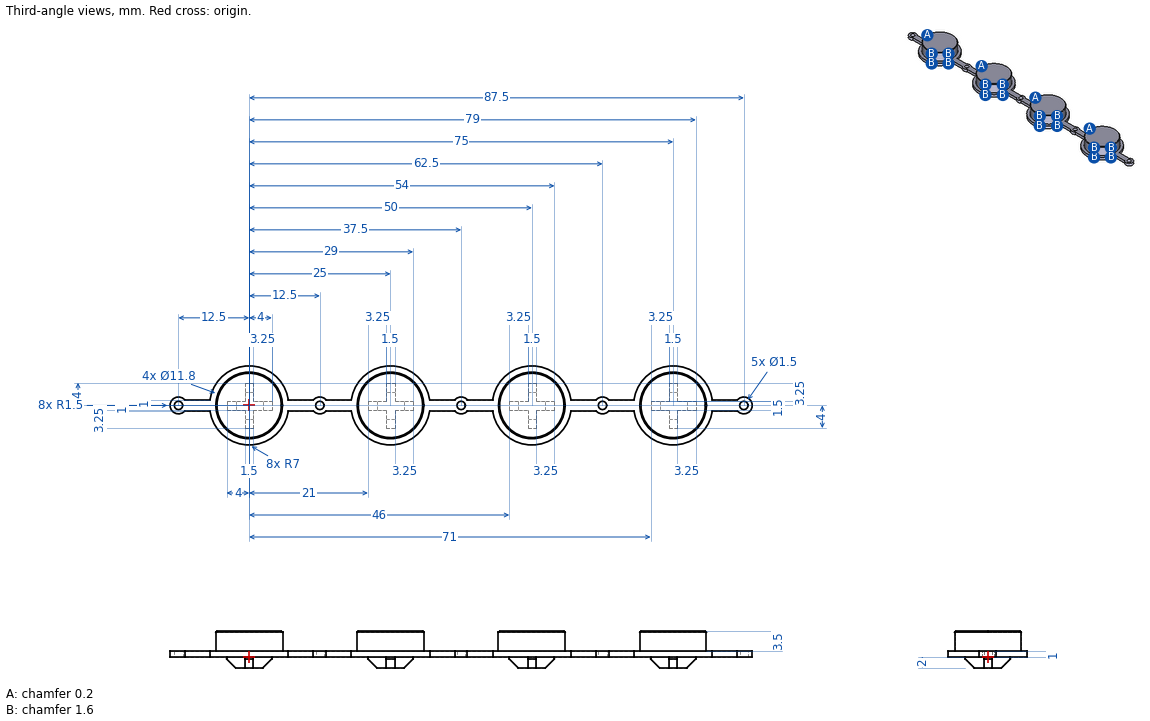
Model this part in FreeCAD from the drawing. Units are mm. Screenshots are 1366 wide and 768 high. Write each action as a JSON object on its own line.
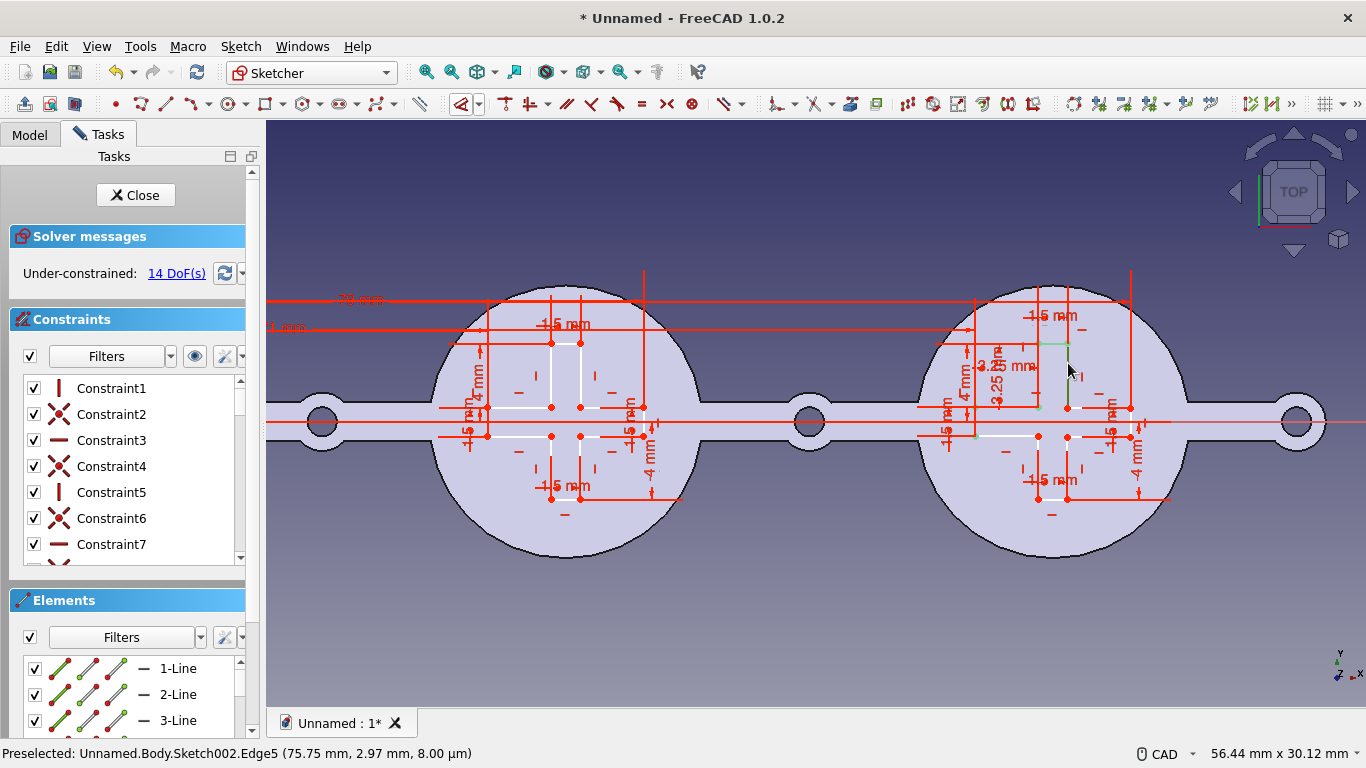
{"action": "key", "text": "i"}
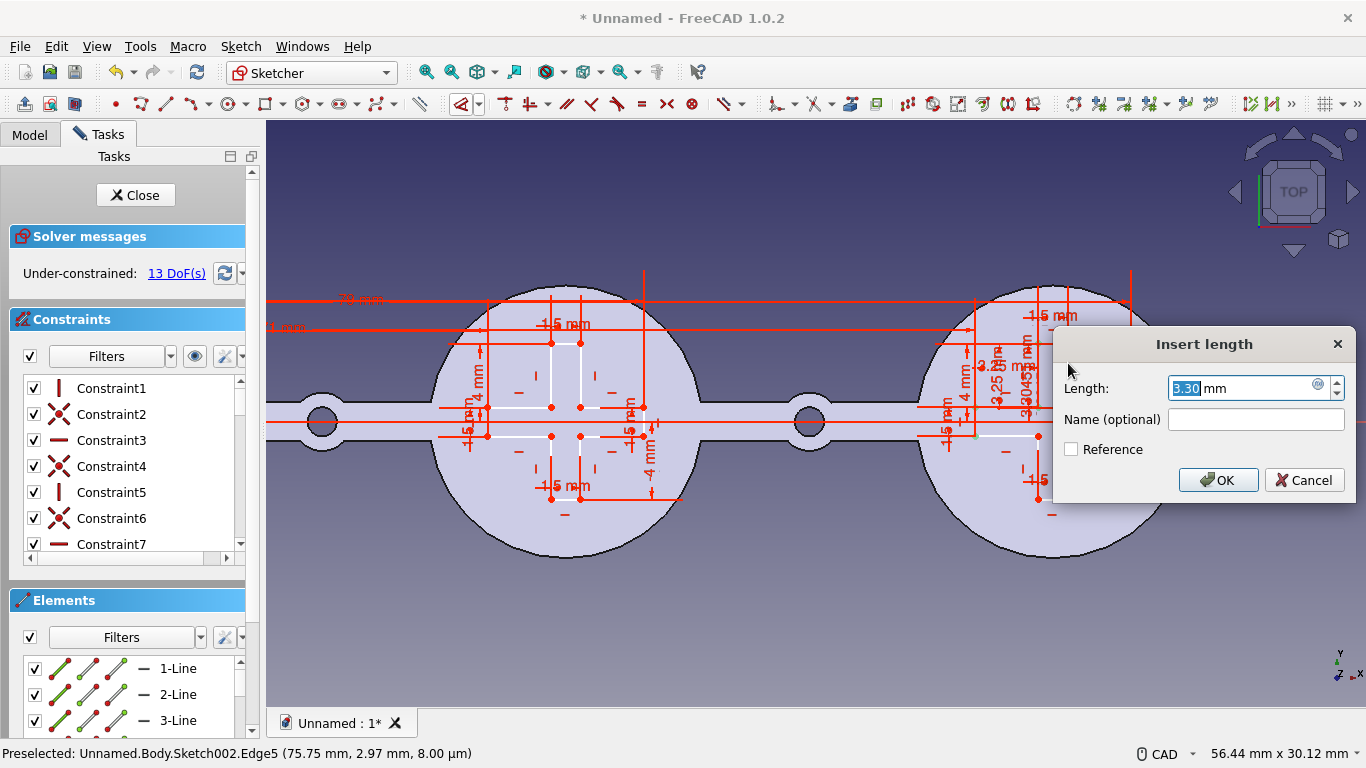
{"action": "type", "text": "3.25"}
{"action": "key", "text": "Return"}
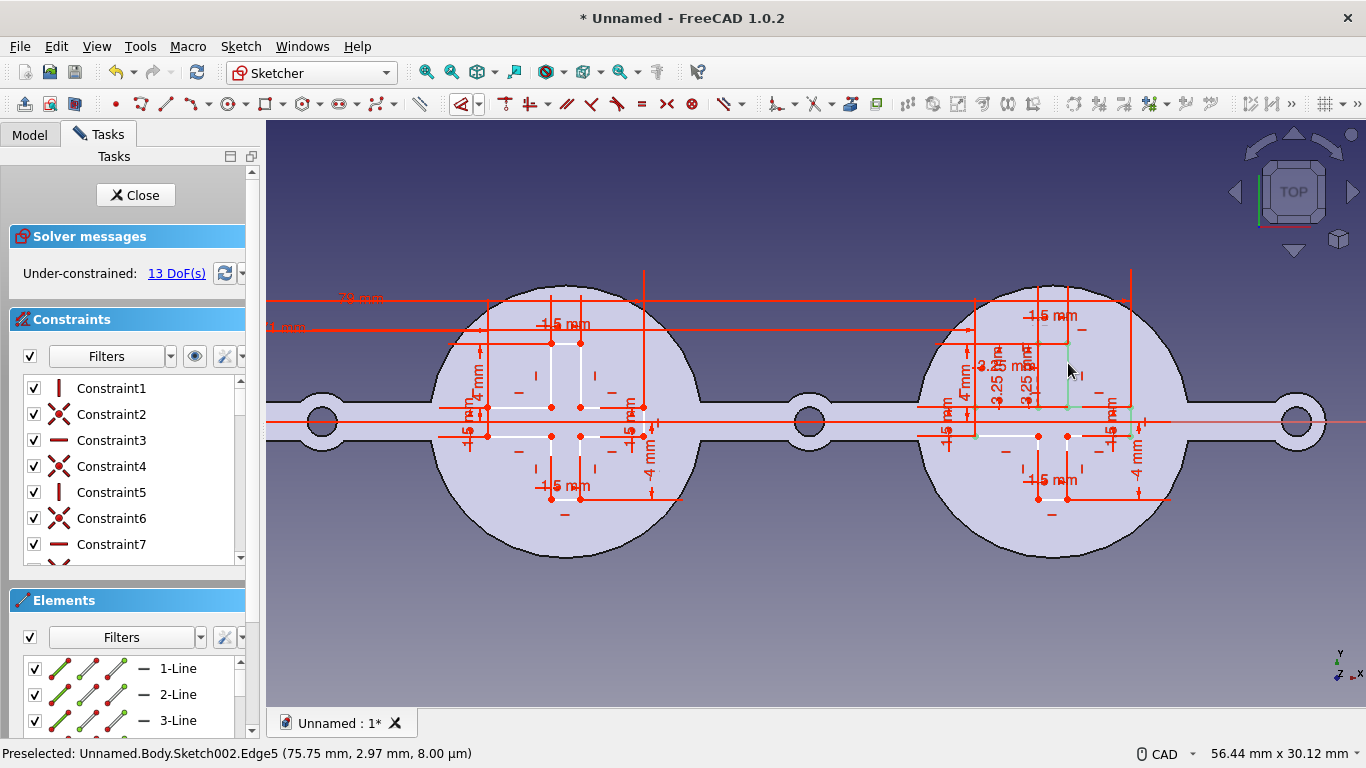
{"action": "left_click", "coordinate": [1087, 436]}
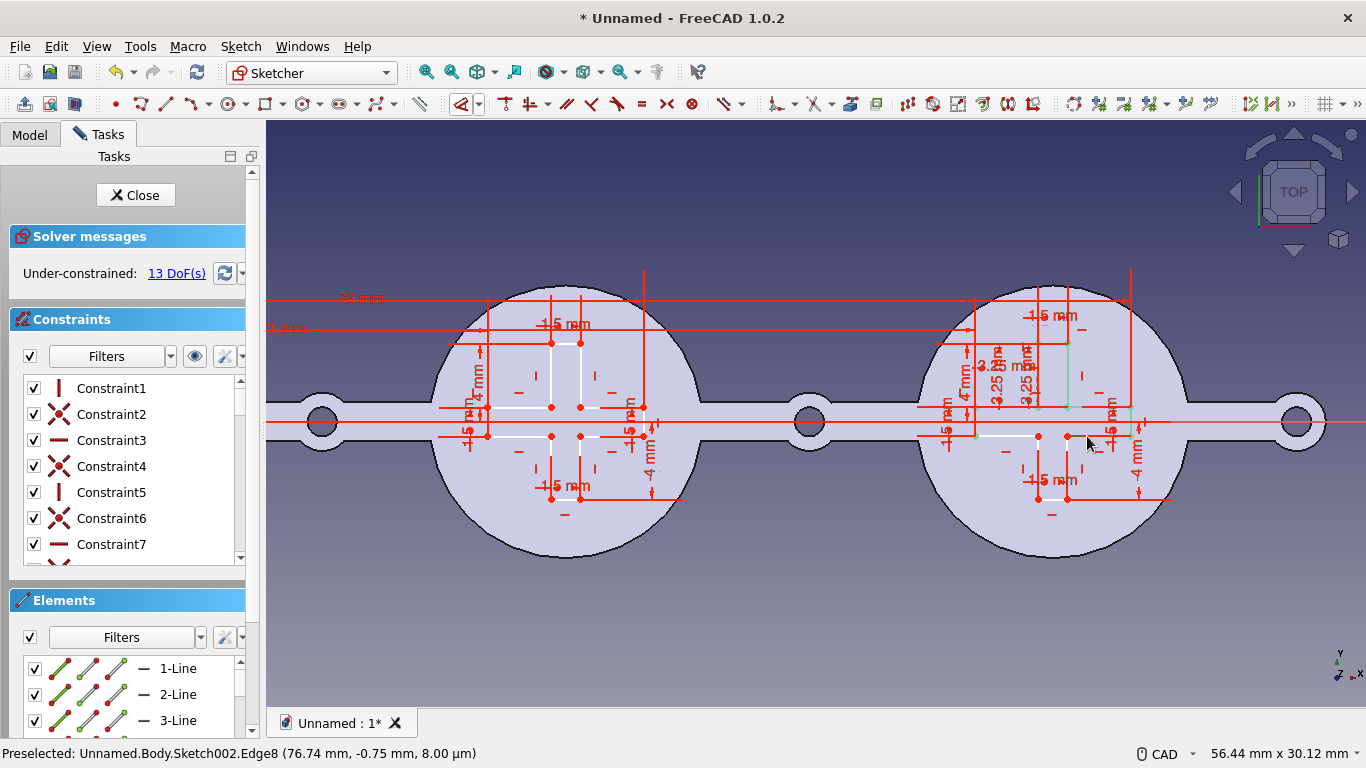
{"action": "key", "text": "l"}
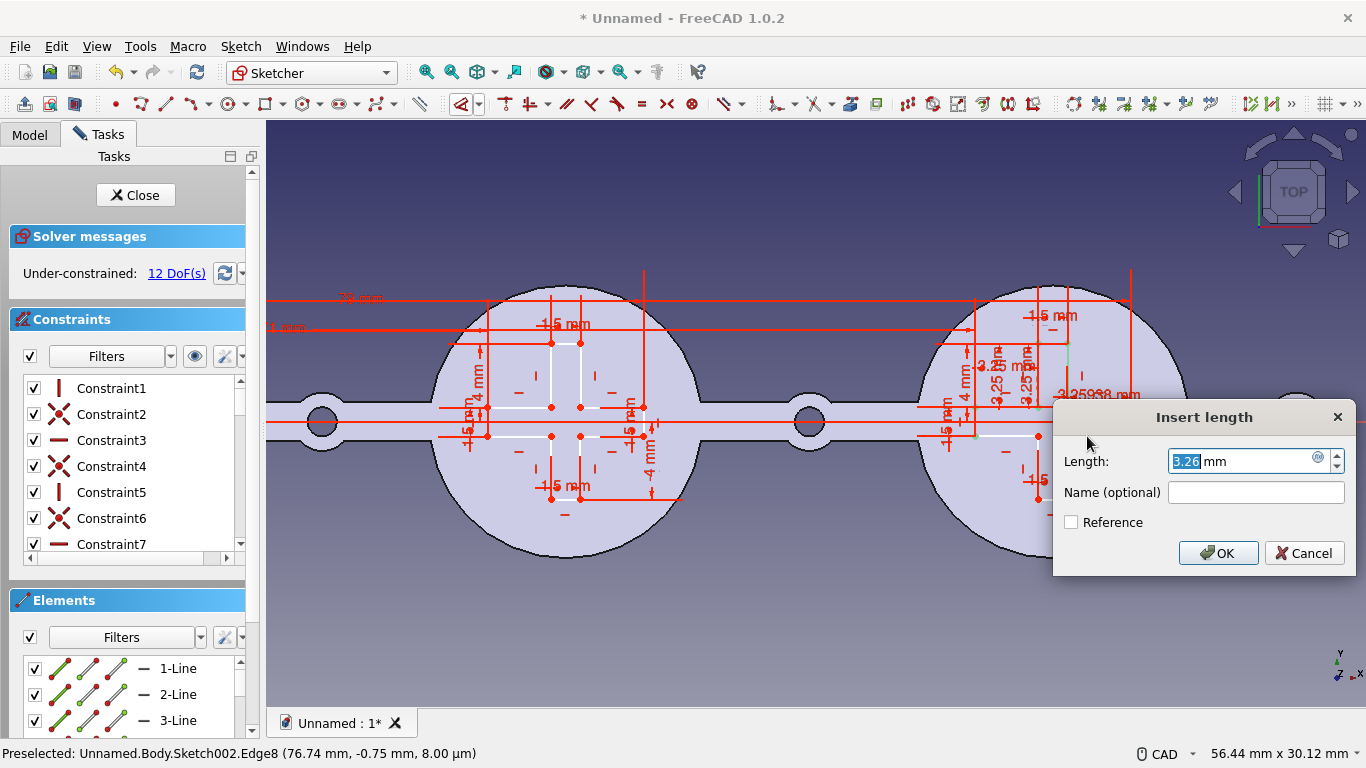
{"action": "type", "text": "3.25"}
{"action": "key", "text": "Return"}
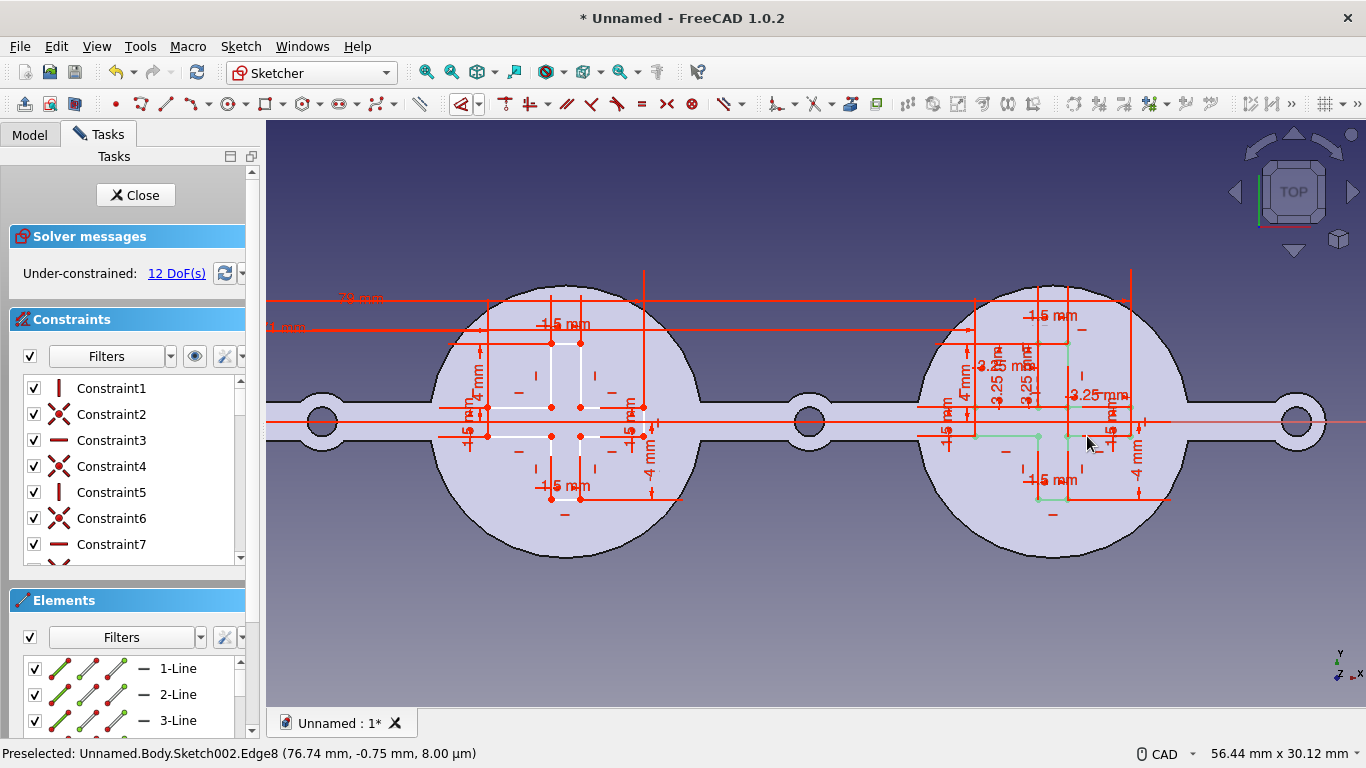
{"action": "left_click", "coordinate": [507, 408]}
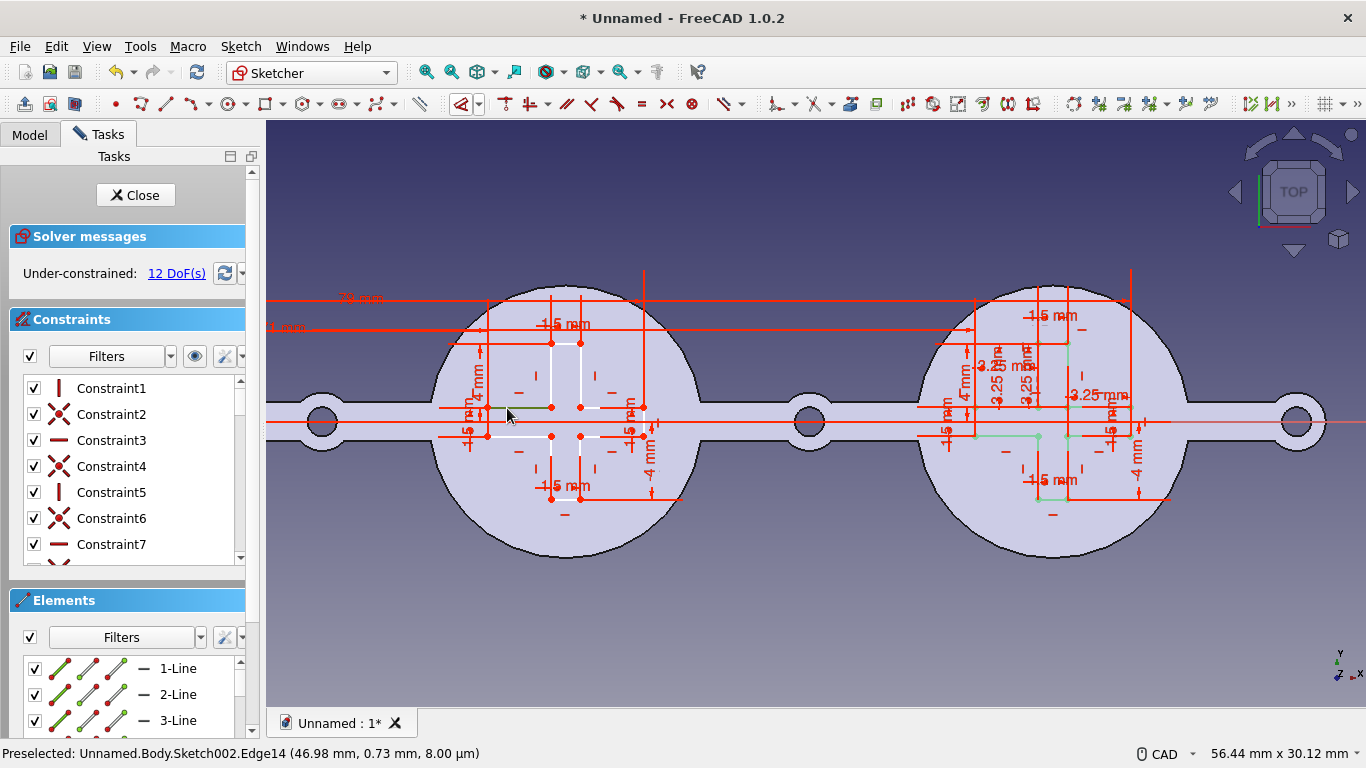
{"action": "key", "text": "l"}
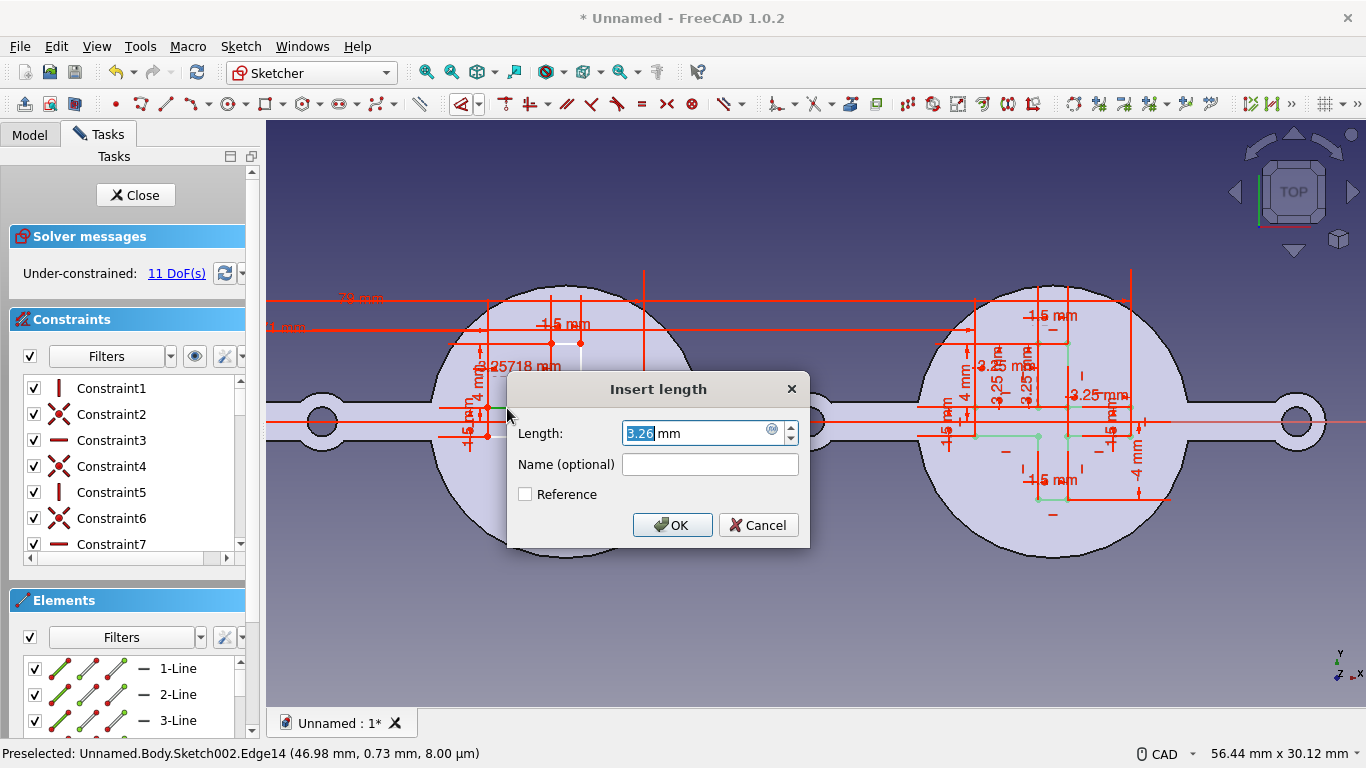
{"action": "type", "text": "3.25"}
{"action": "key", "text": "Return"}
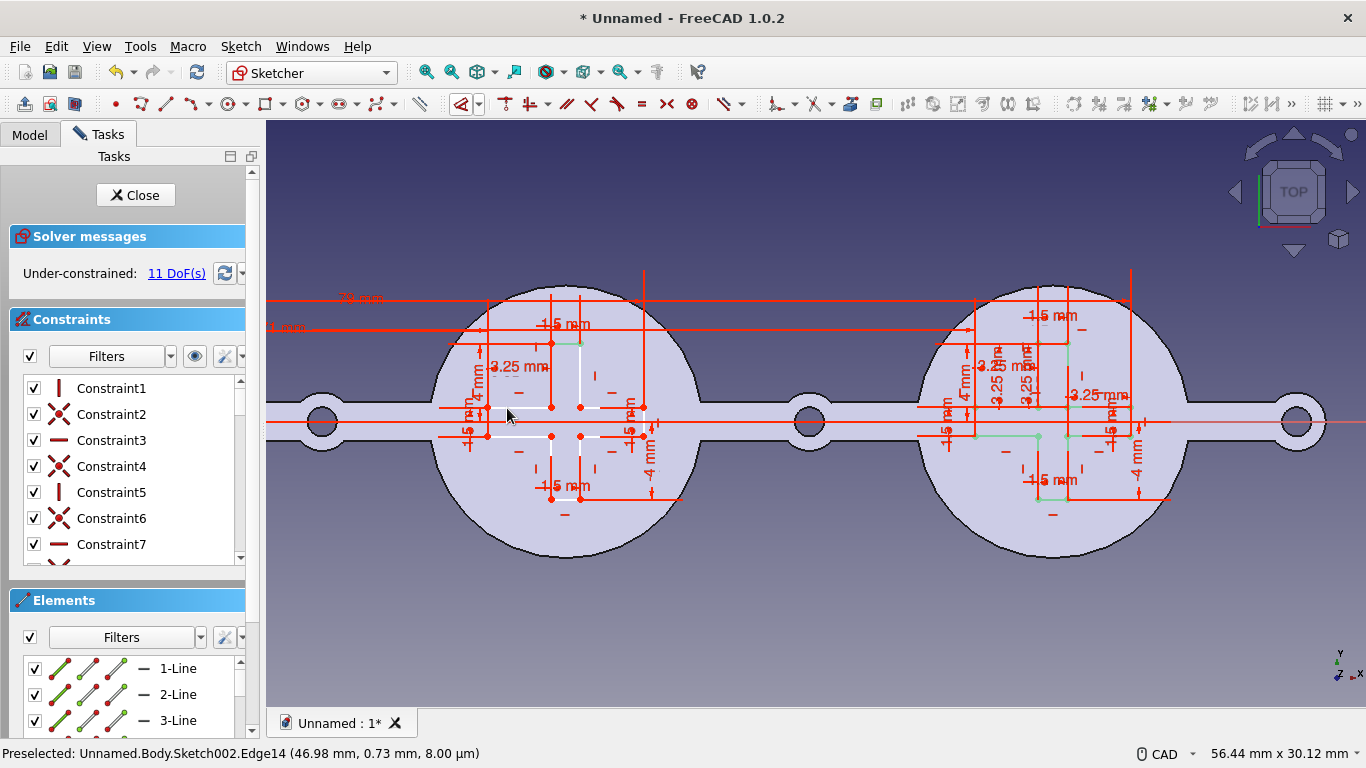
{"action": "left_click", "coordinate": [551, 389]}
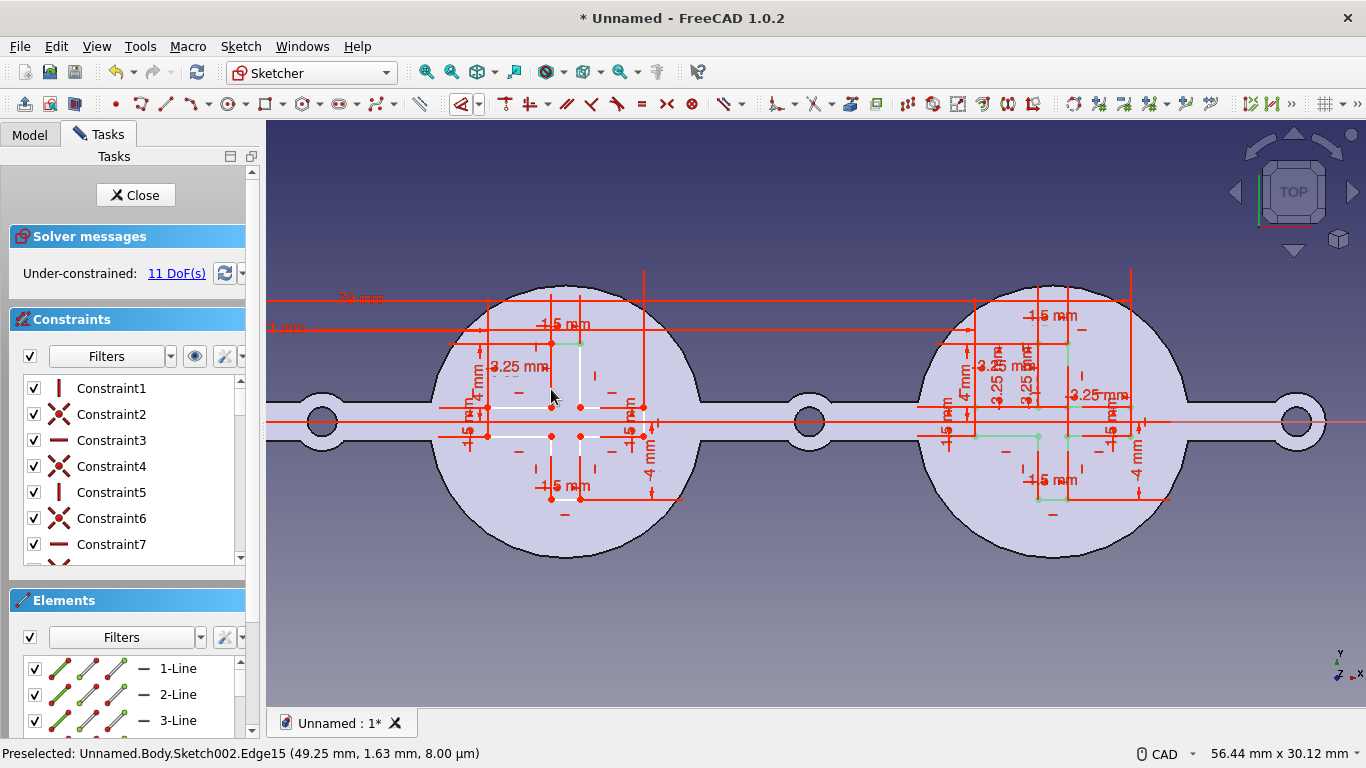
{"action": "left_click", "coordinate": [478, 104]}